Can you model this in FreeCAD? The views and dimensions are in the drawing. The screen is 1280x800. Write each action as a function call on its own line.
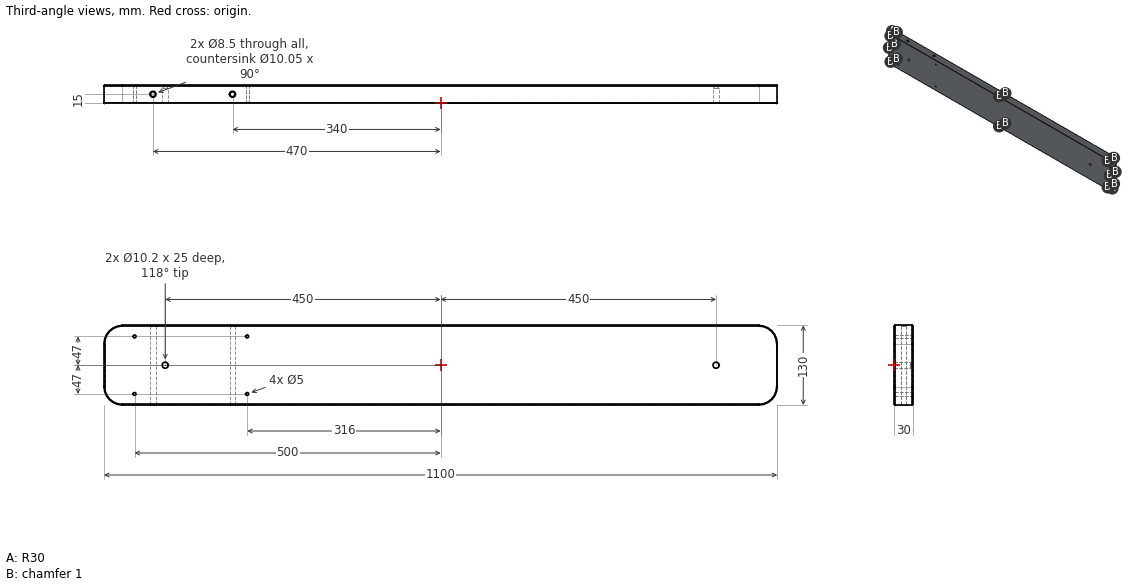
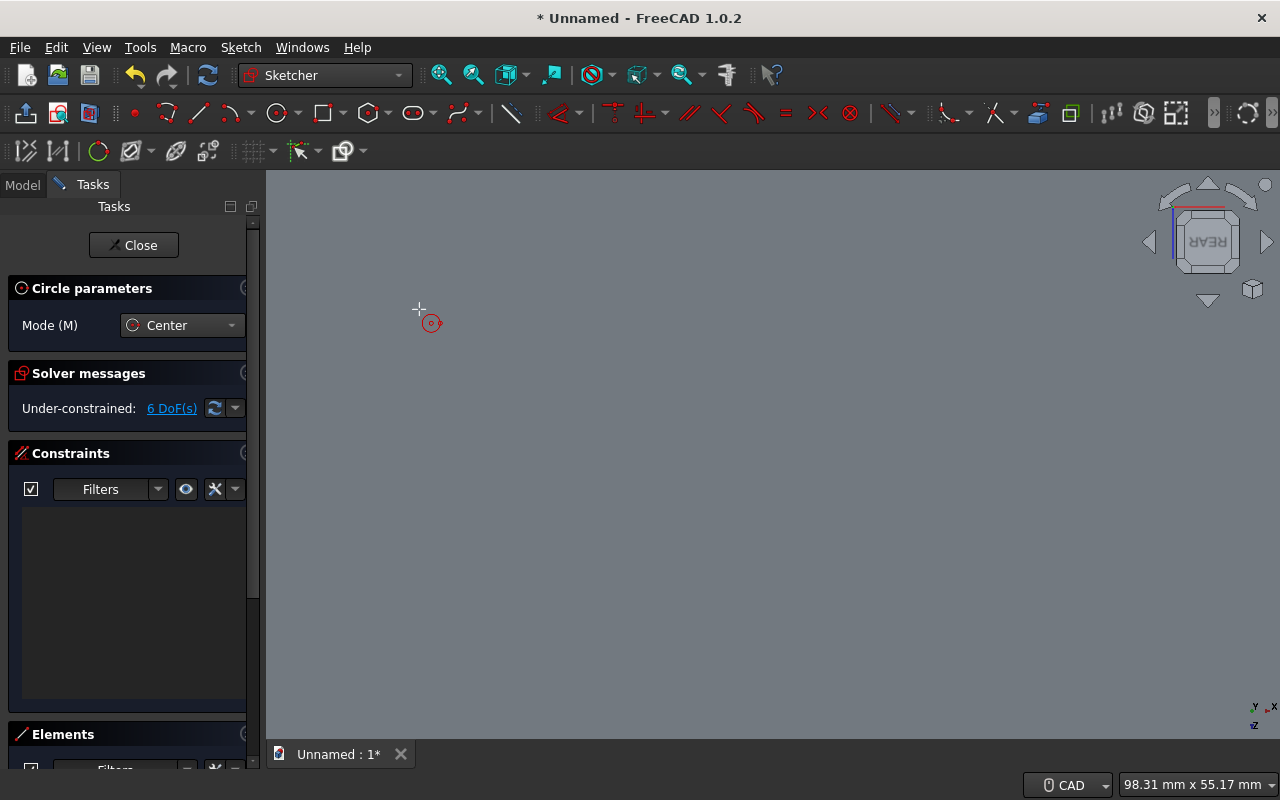
click(420, 309)
click(438, 291)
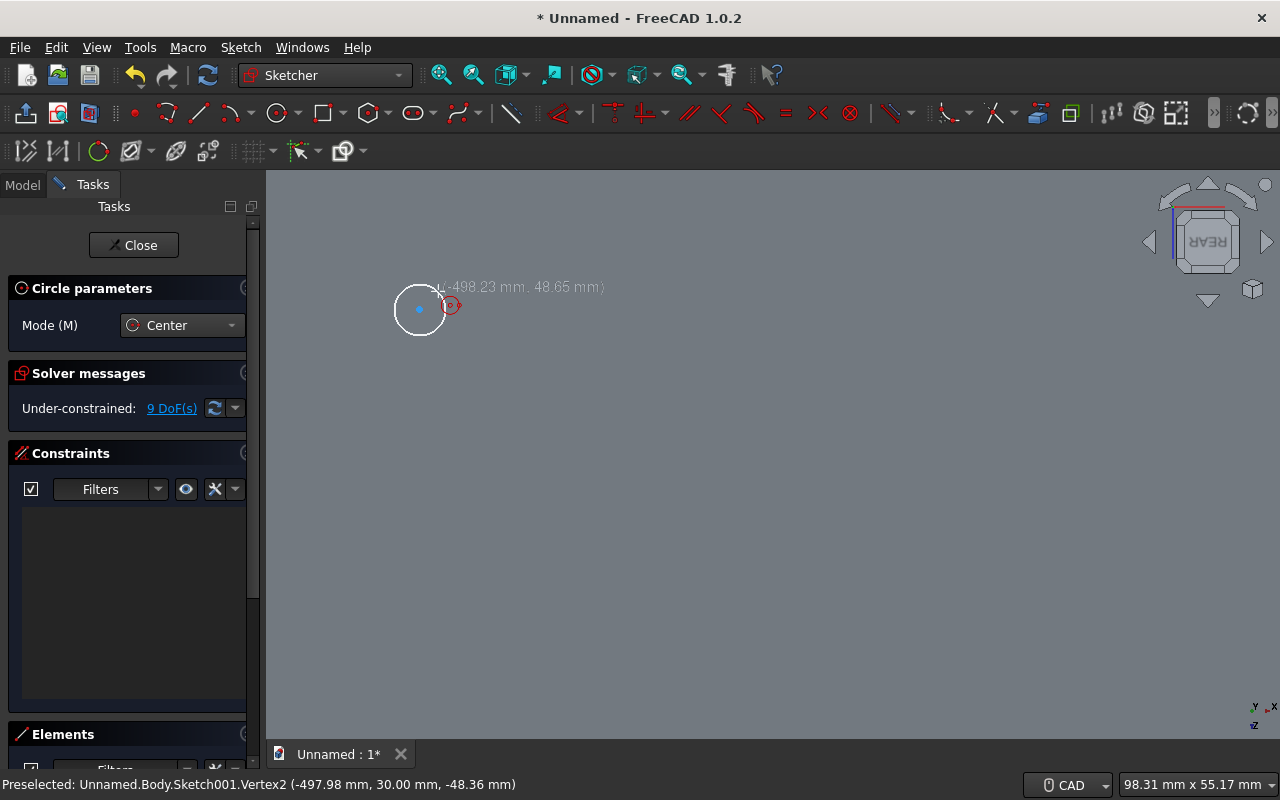
scroll(418, 308, down, 6)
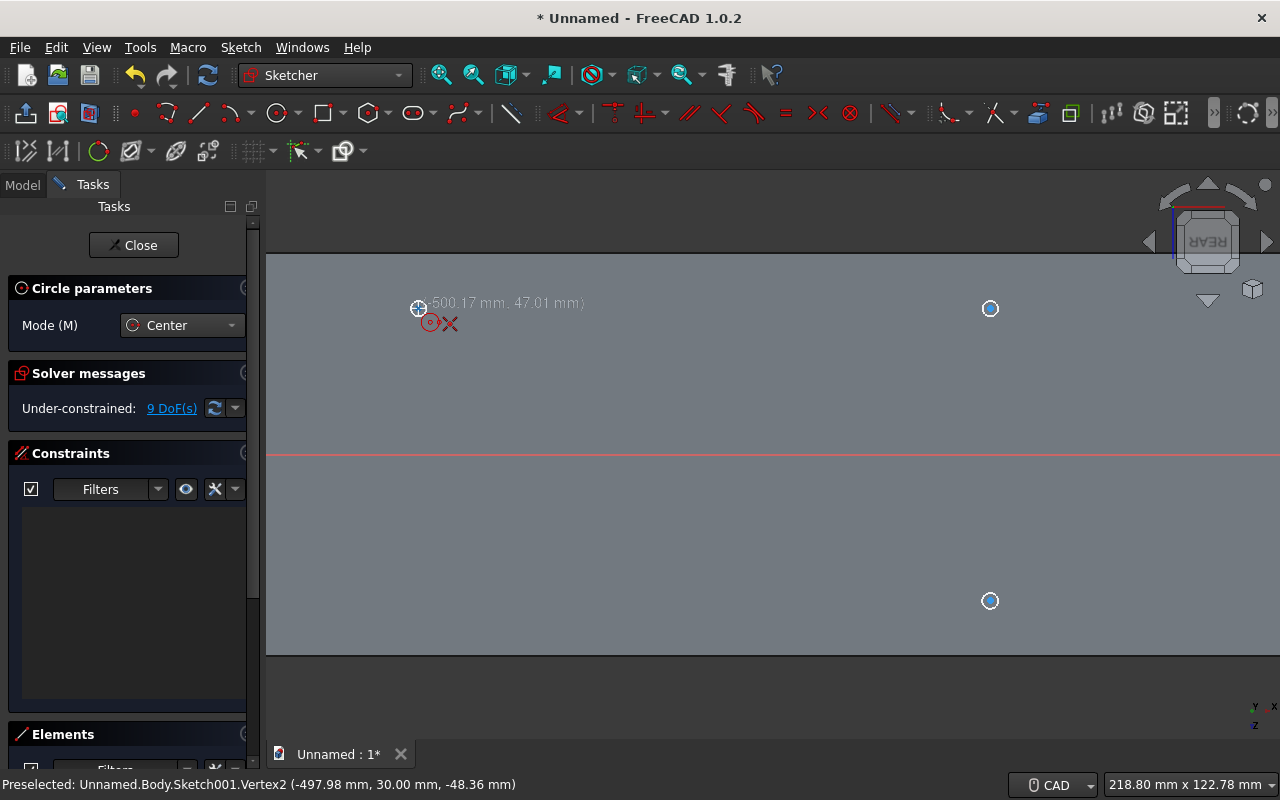
scroll(419, 601, up, 6)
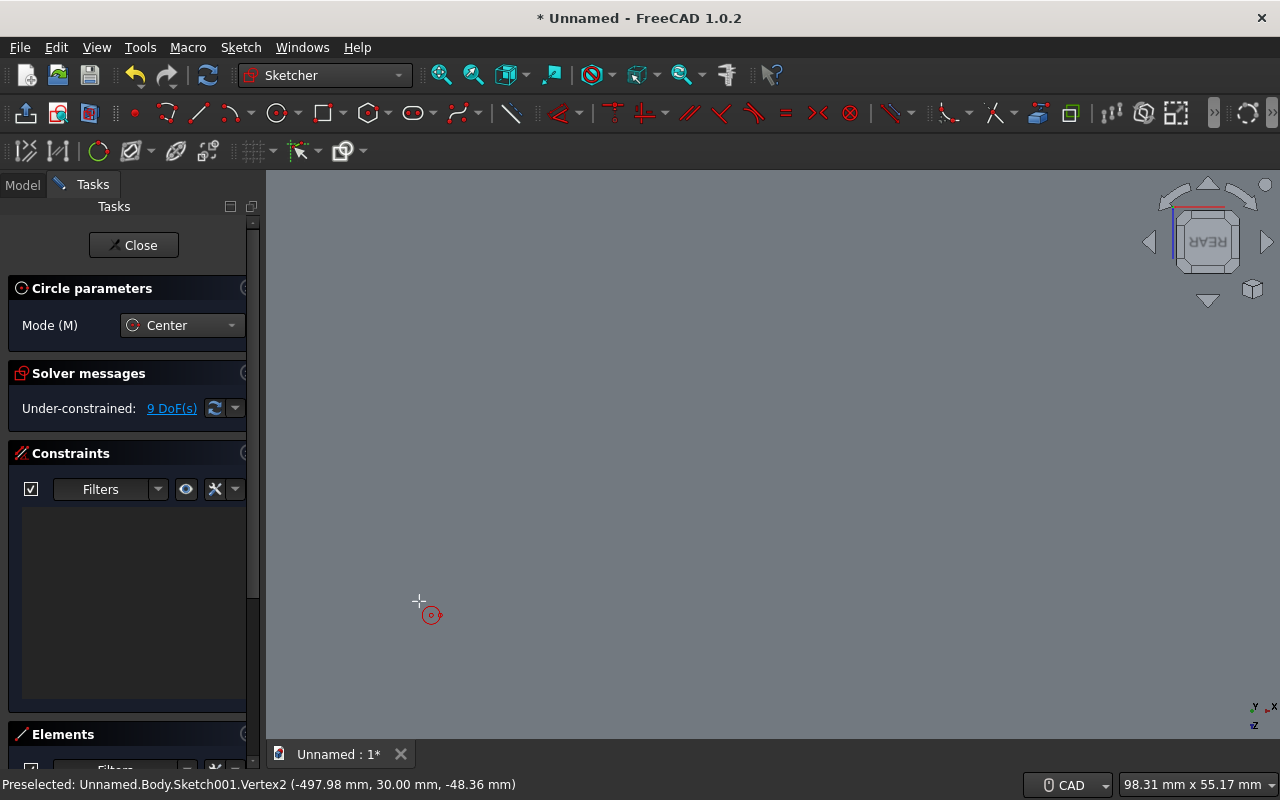
click(417, 598)
click(436, 579)
key(Escape)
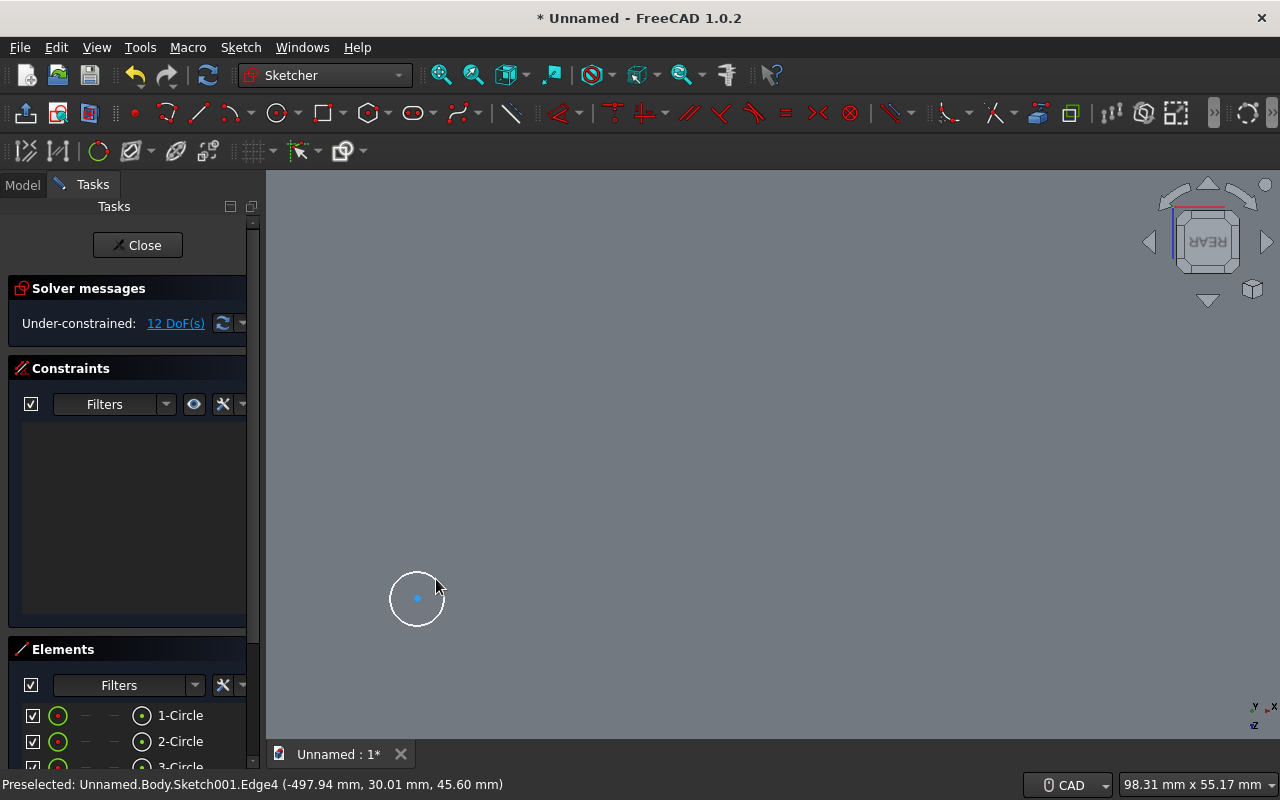
scroll(419, 602, down, 6)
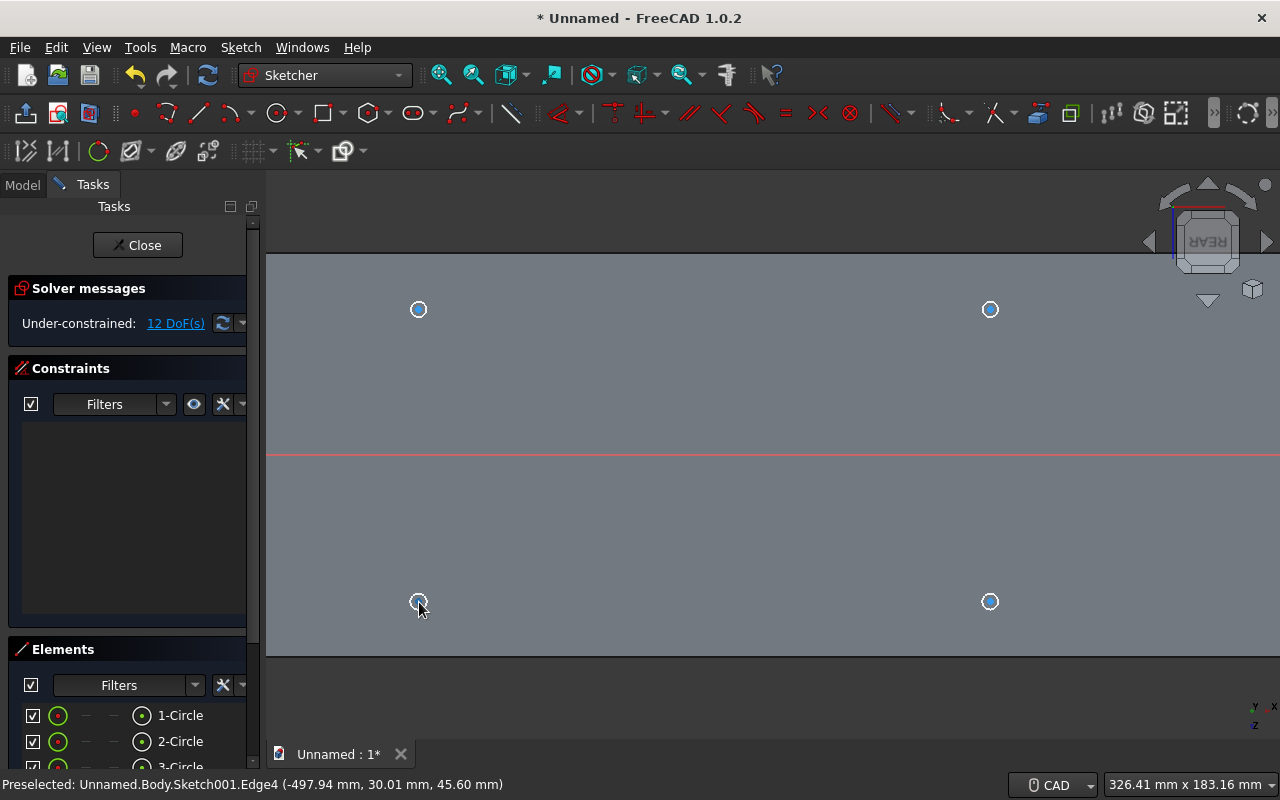
scroll(996, 304, up, 3)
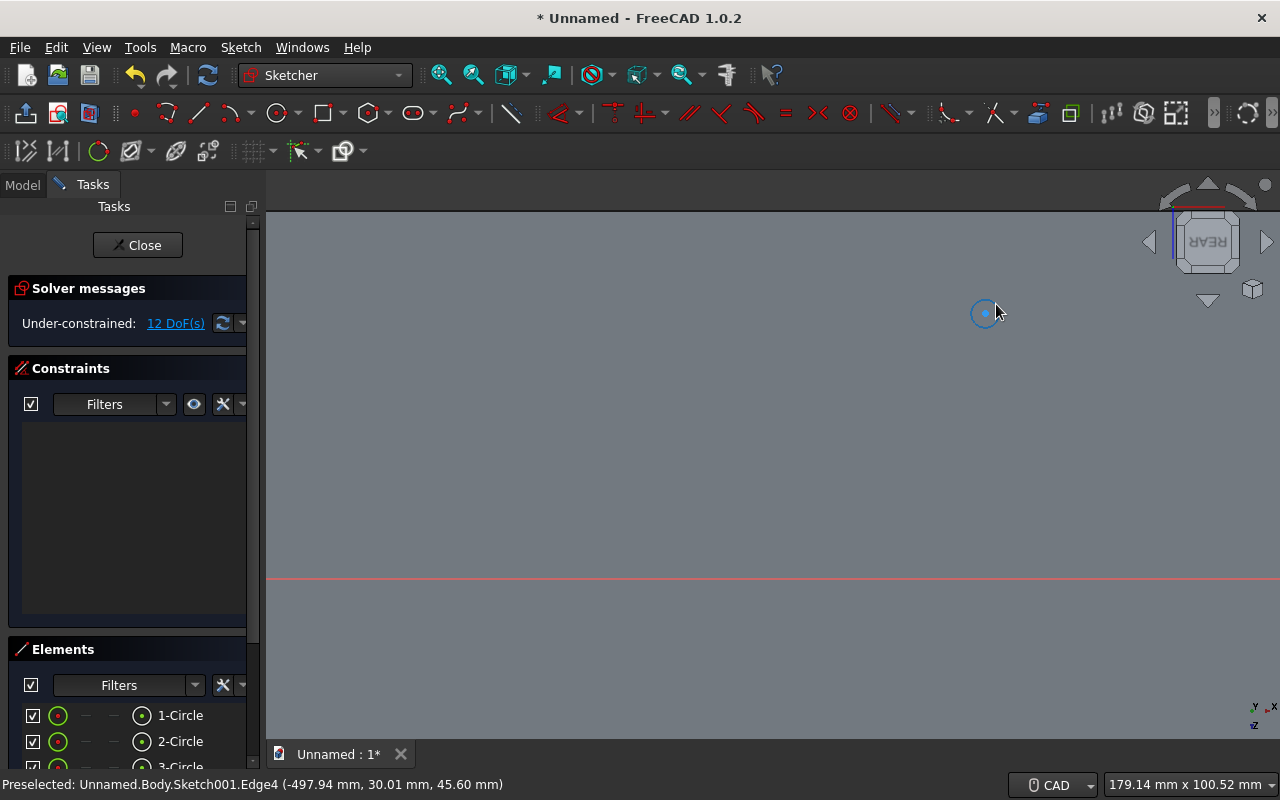
click(995, 304)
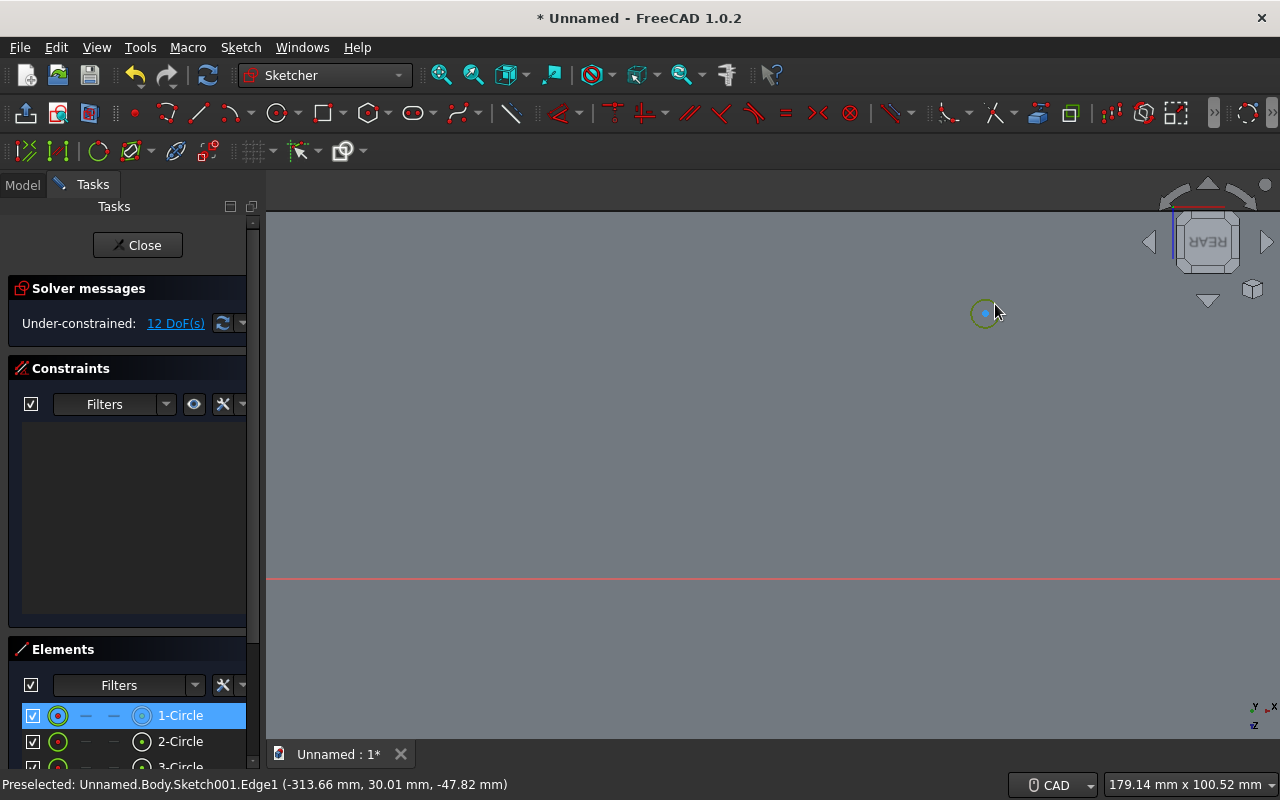
scroll(997, 303, down, 3)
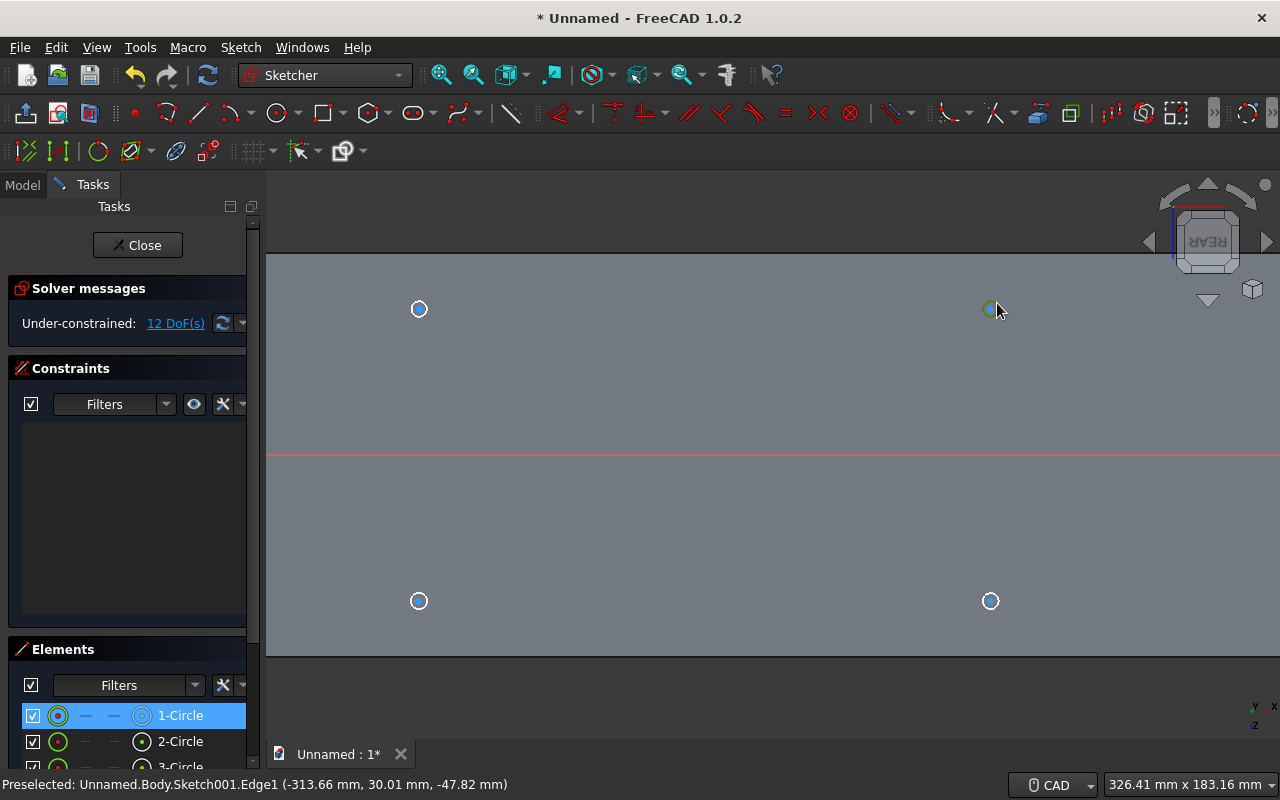
scroll(996, 596, up, 3)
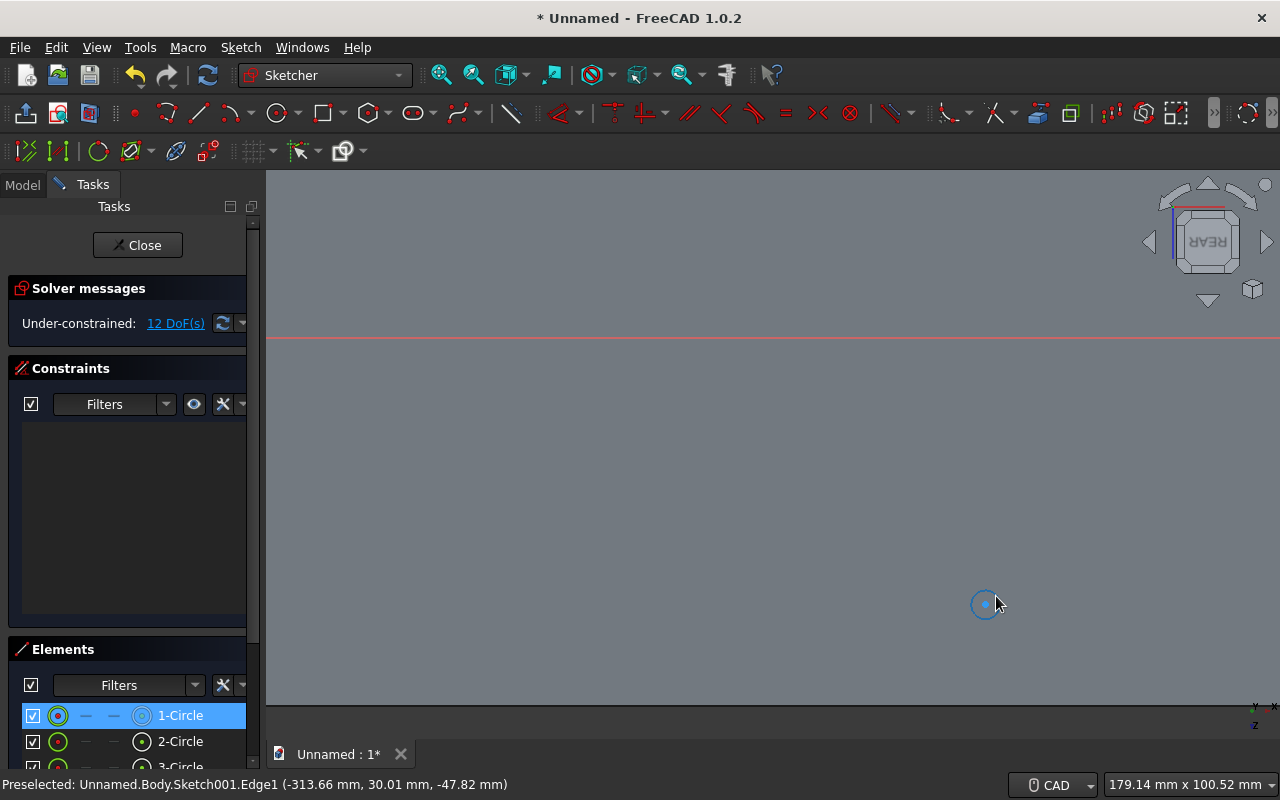
click(996, 595)